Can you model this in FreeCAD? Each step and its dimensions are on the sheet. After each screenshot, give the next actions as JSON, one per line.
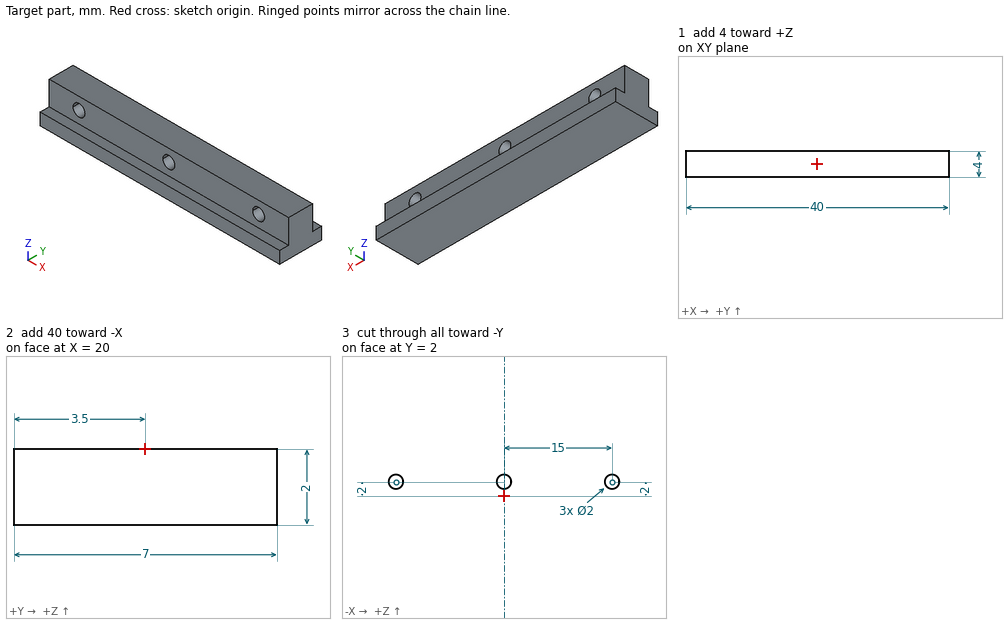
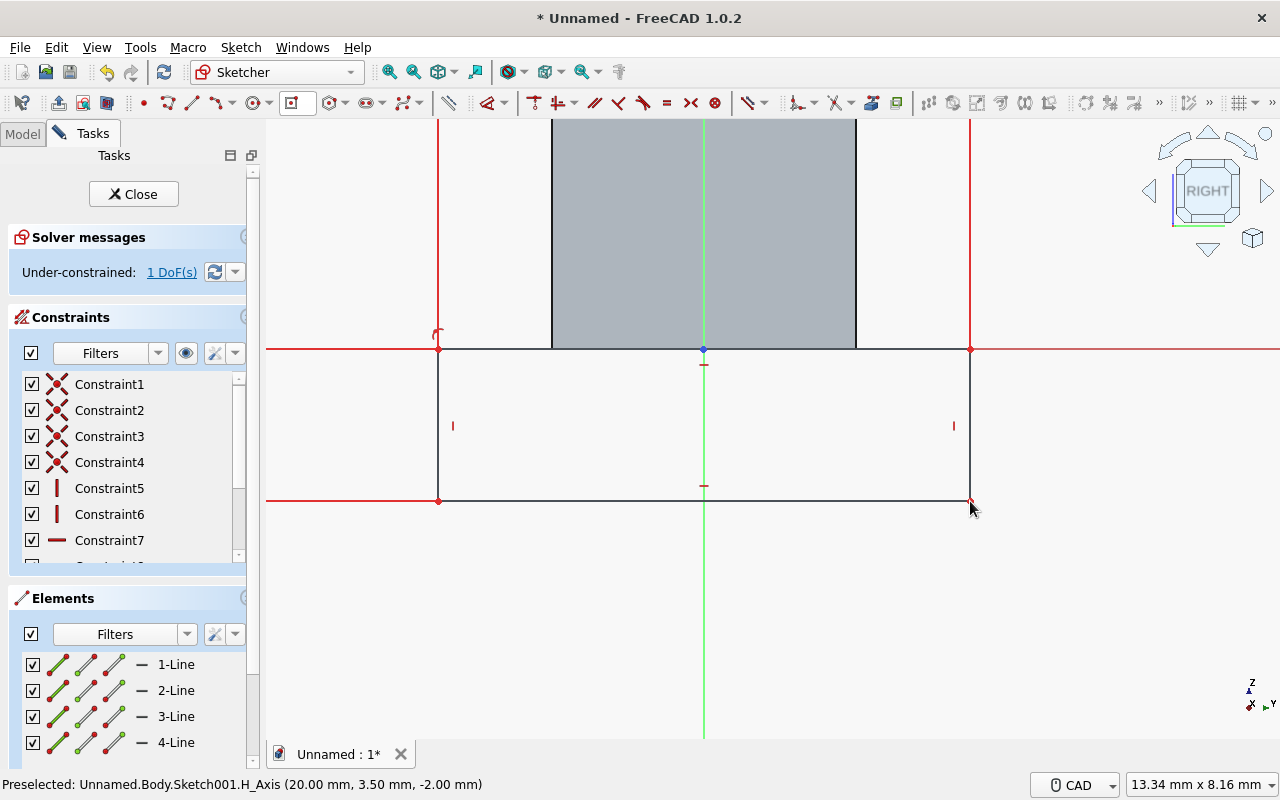
{"action": "key", "text": "d"}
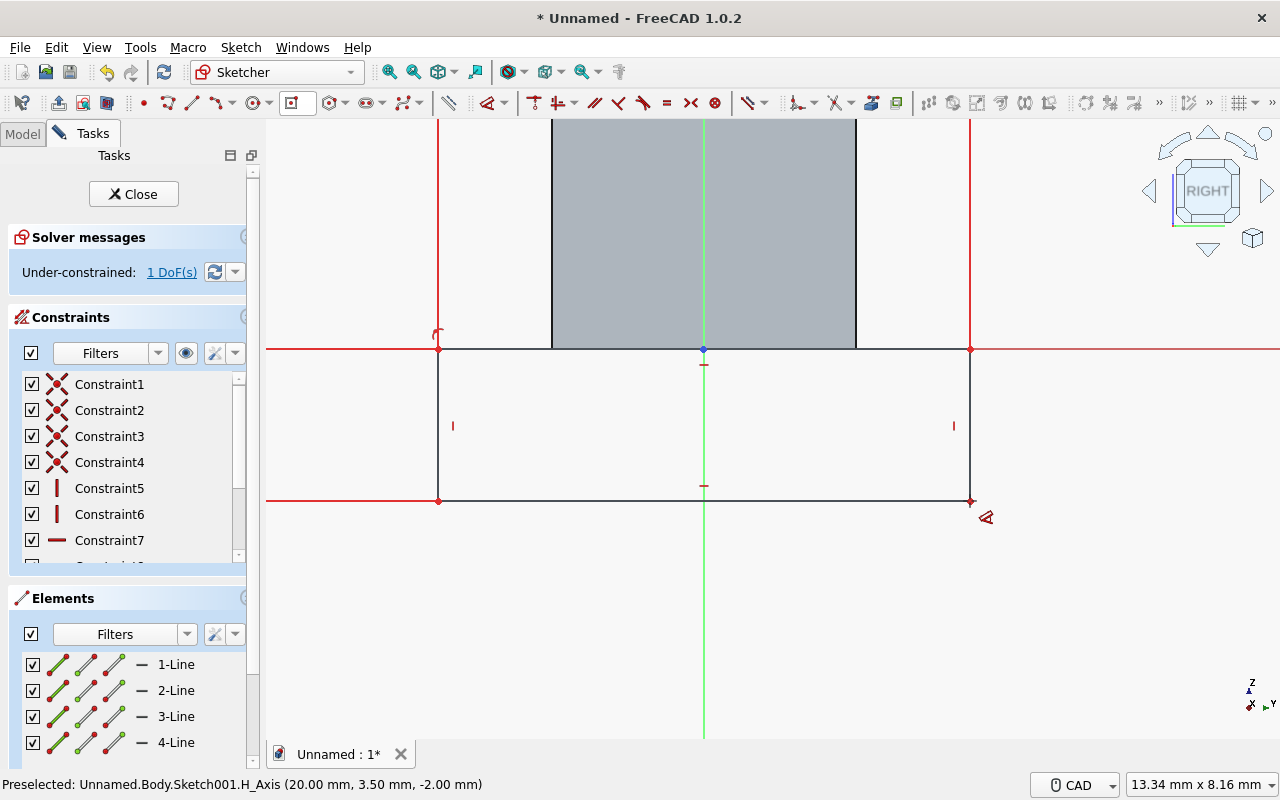
{"action": "left_click", "coordinate": [438, 349]}
{"action": "left_click", "coordinate": [571, 315]}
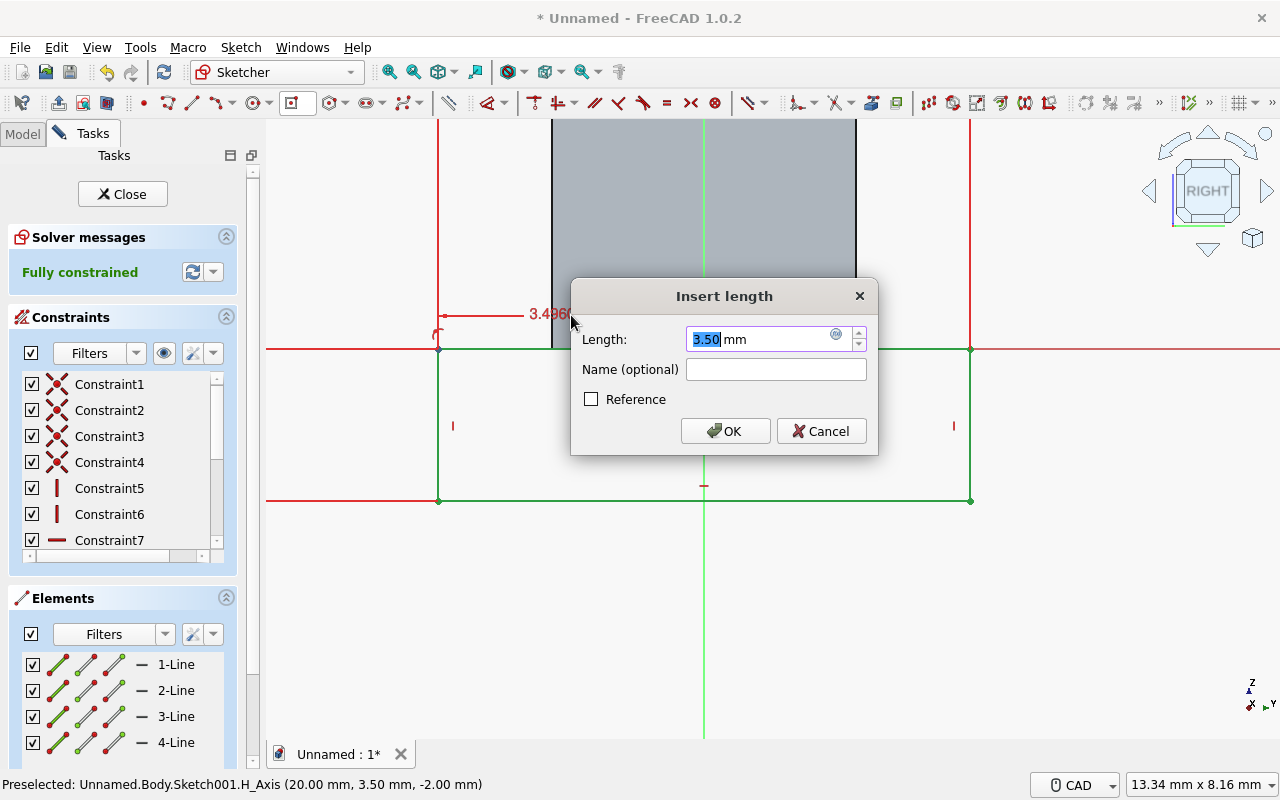
{"action": "type", "text": "3.5"}
{"action": "key", "text": "Return"}
{"action": "key", "text": "Escape"}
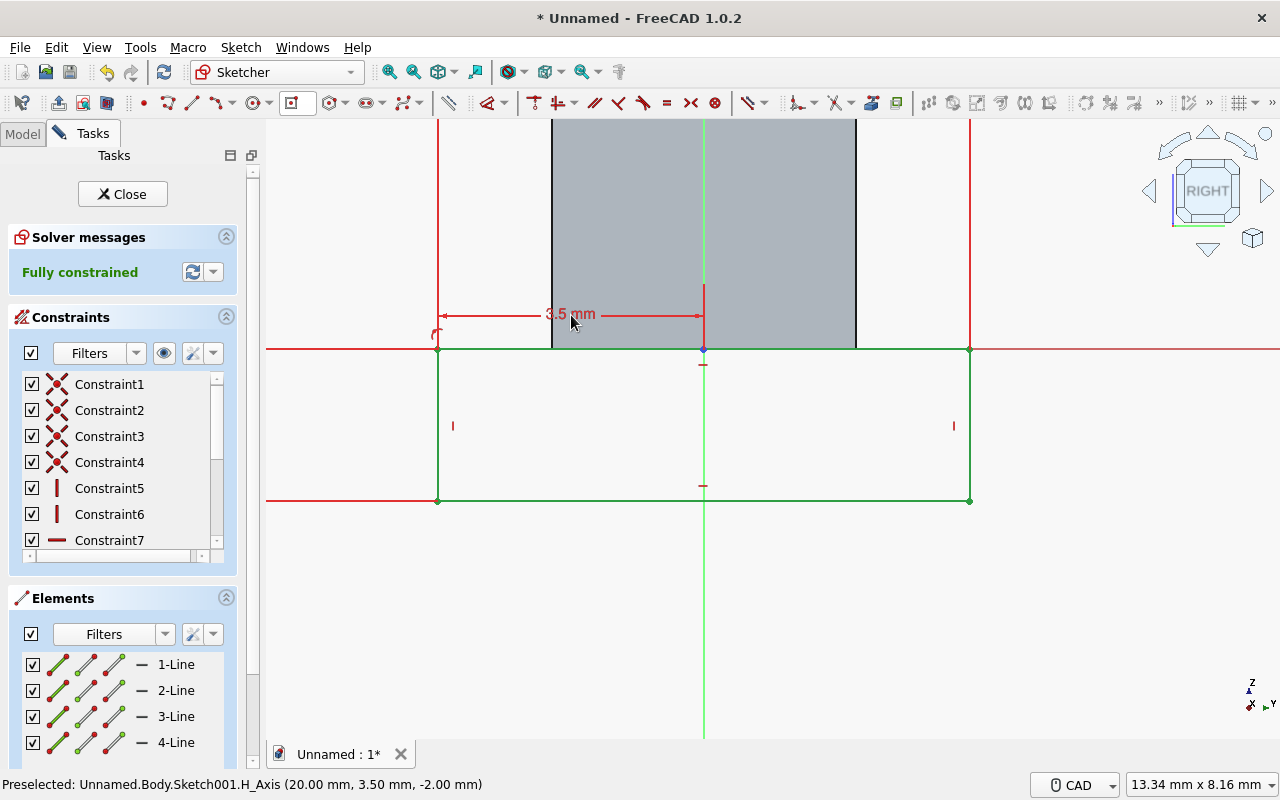
{"action": "left_click", "coordinate": [123, 194]}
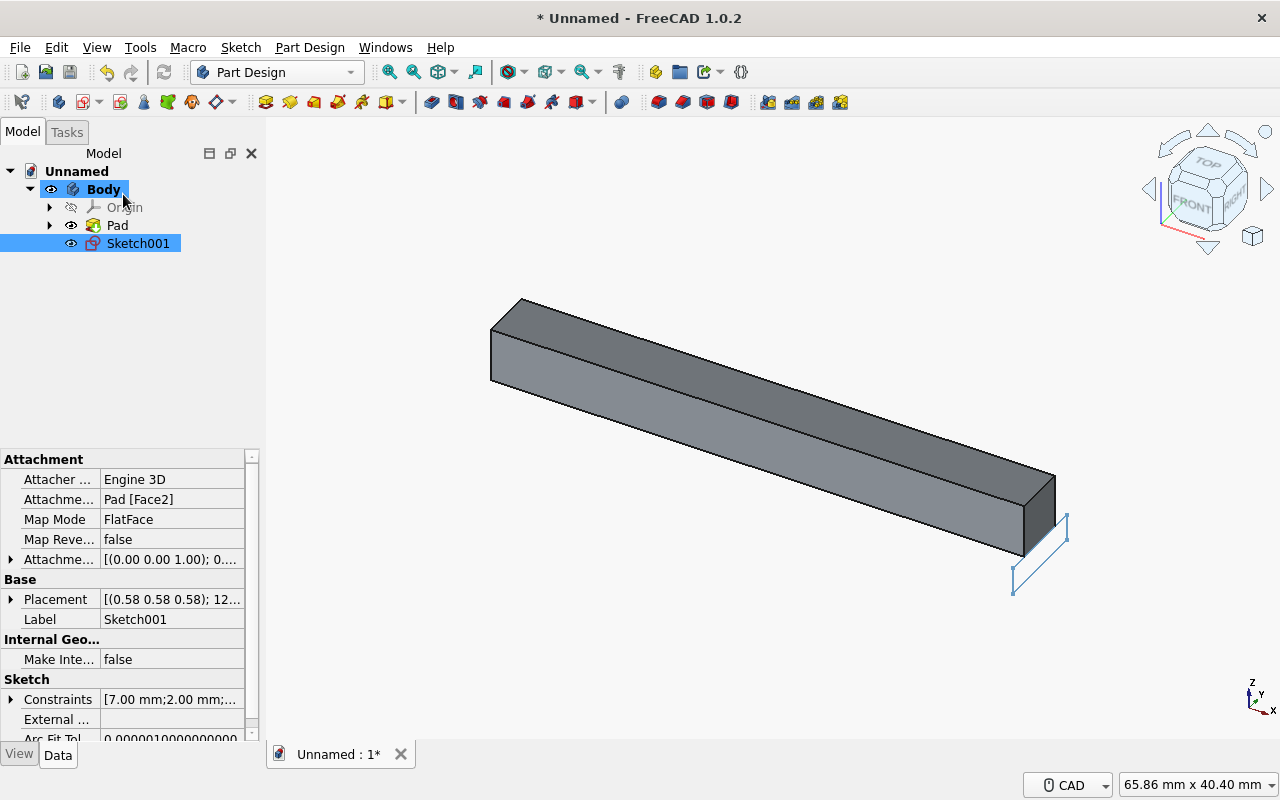
{"action": "left_click", "coordinate": [266, 102]}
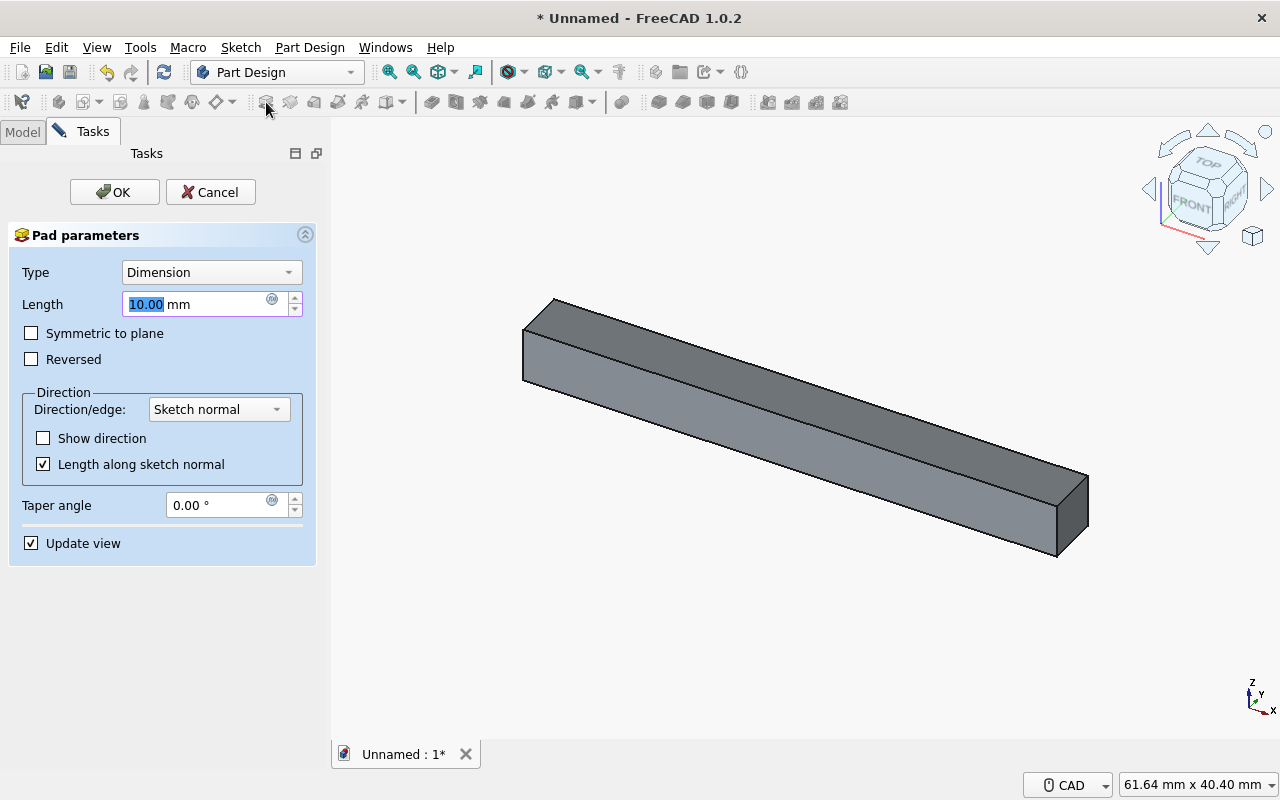
{"action": "type", "text": "40"}
{"action": "key", "text": "Tab"}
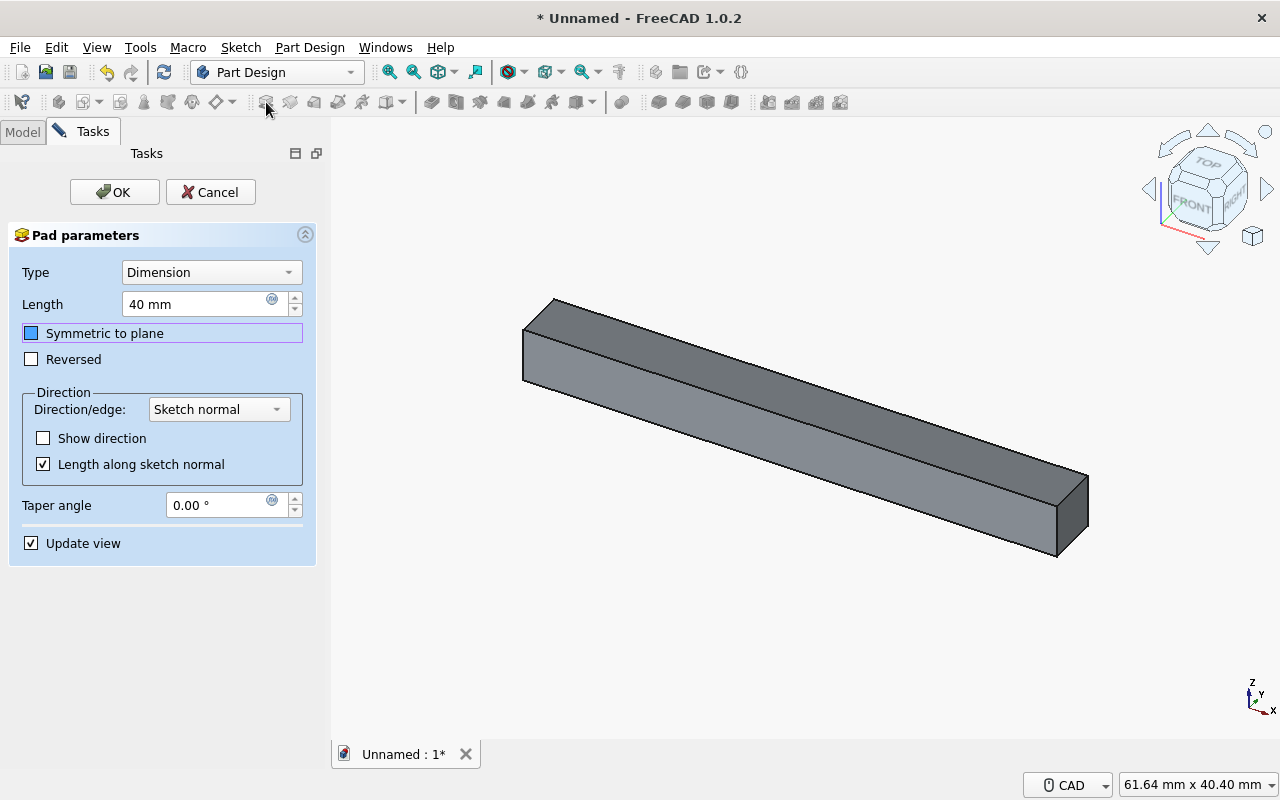
{"action": "left_click", "coordinate": [30, 359]}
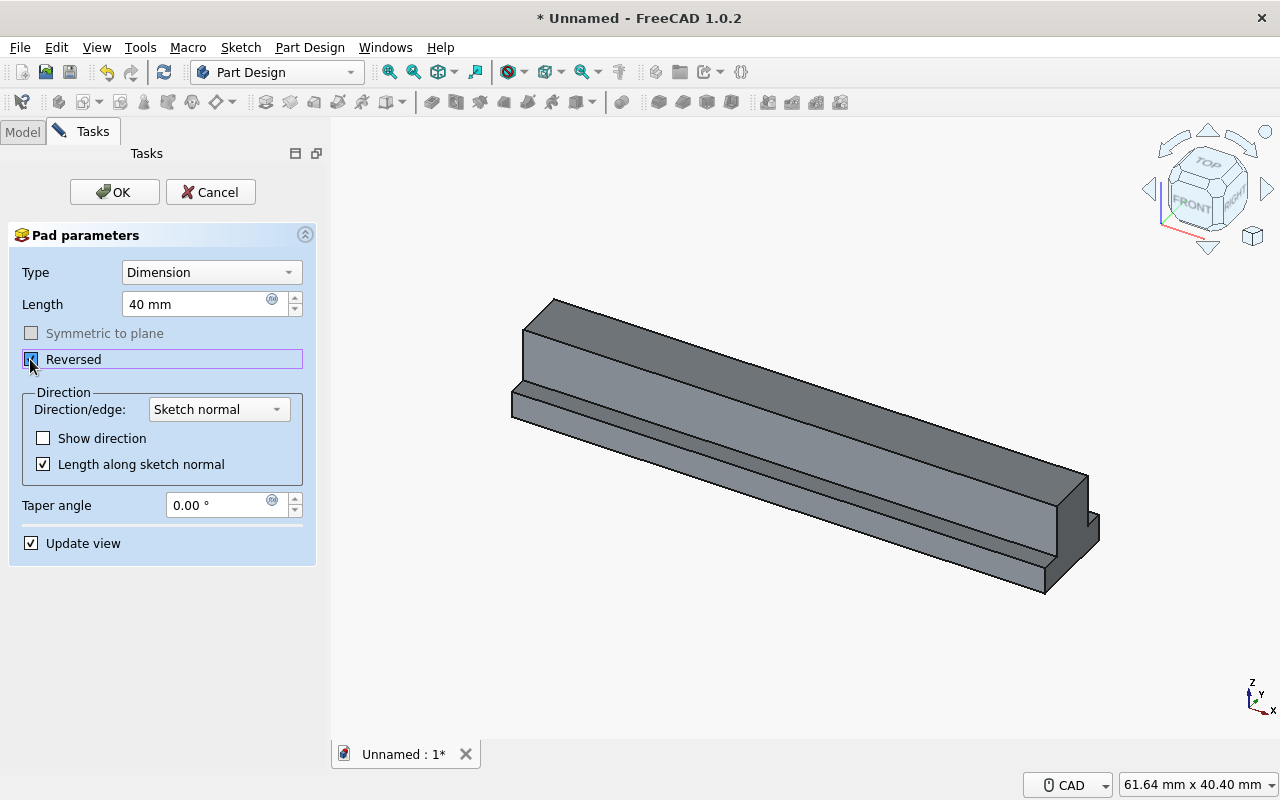
{"action": "left_click", "coordinate": [115, 192]}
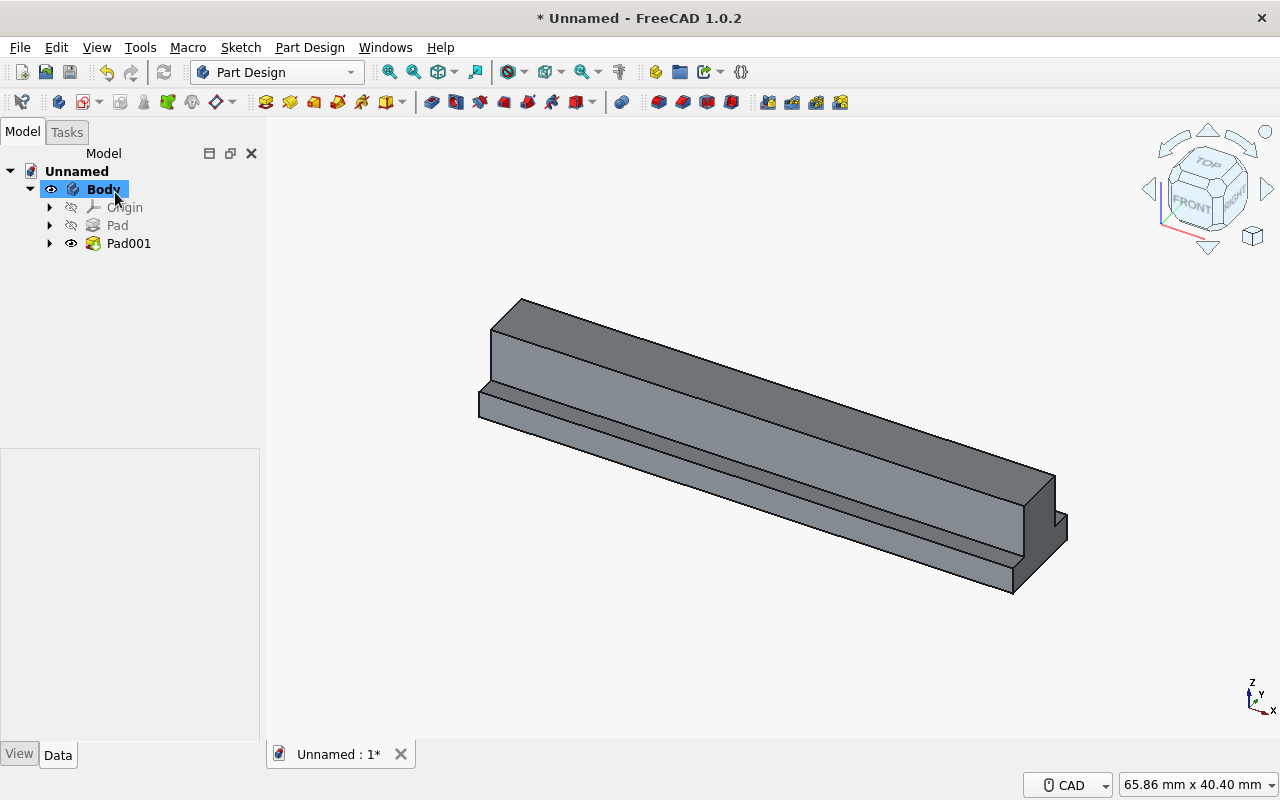
{"action": "key", "text": "4"}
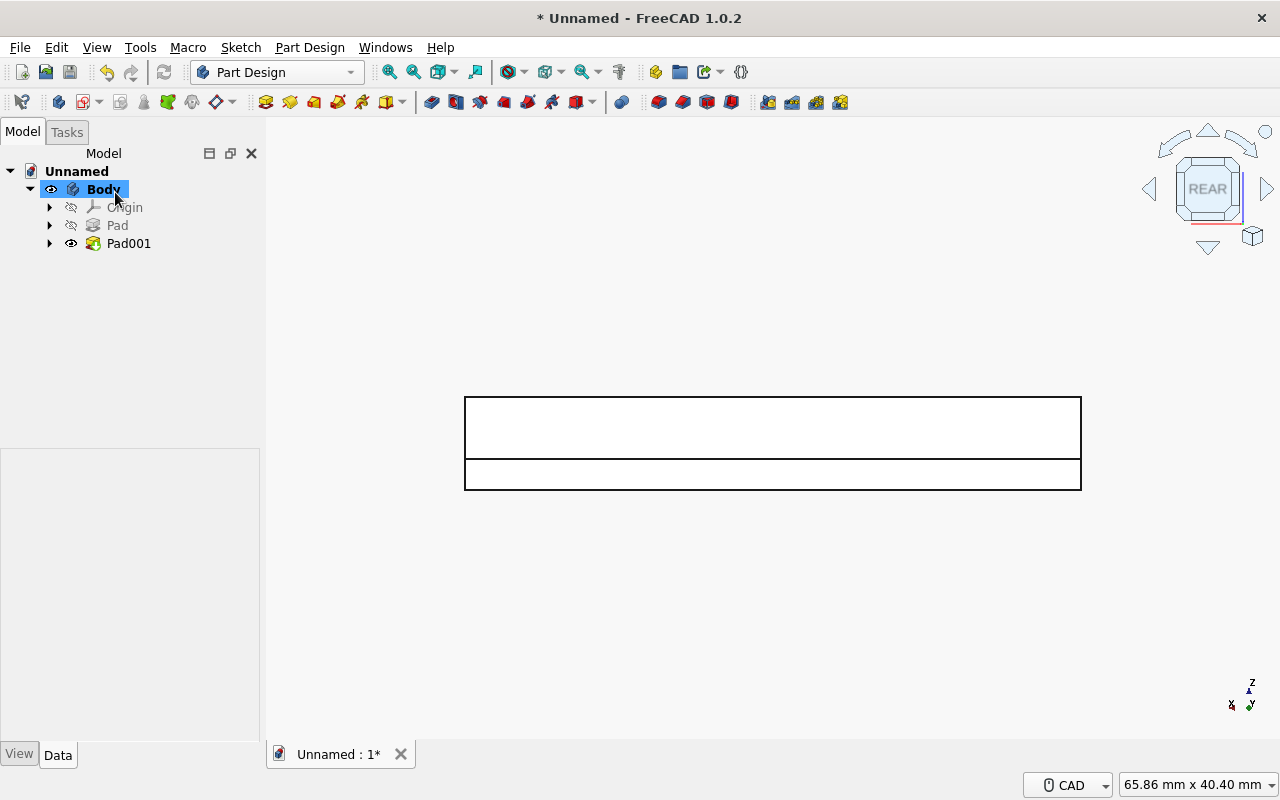
{"action": "left_click", "coordinate": [509, 427]}